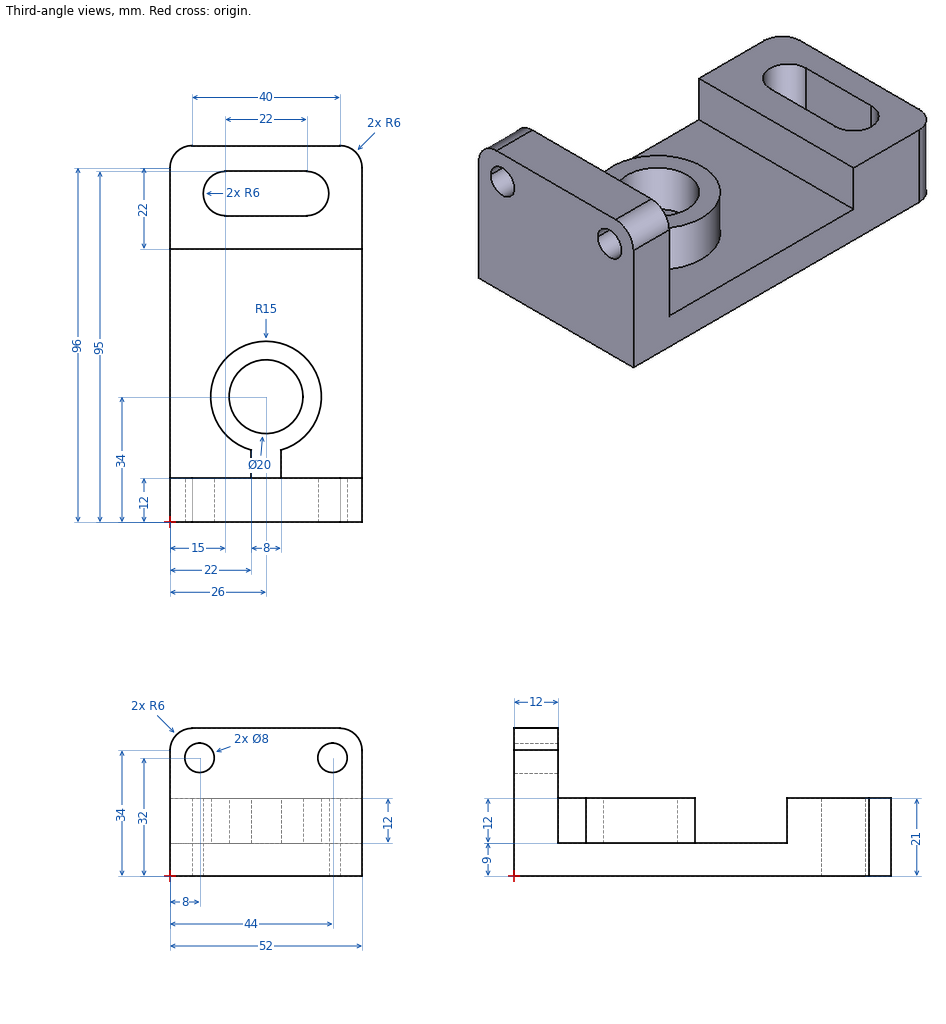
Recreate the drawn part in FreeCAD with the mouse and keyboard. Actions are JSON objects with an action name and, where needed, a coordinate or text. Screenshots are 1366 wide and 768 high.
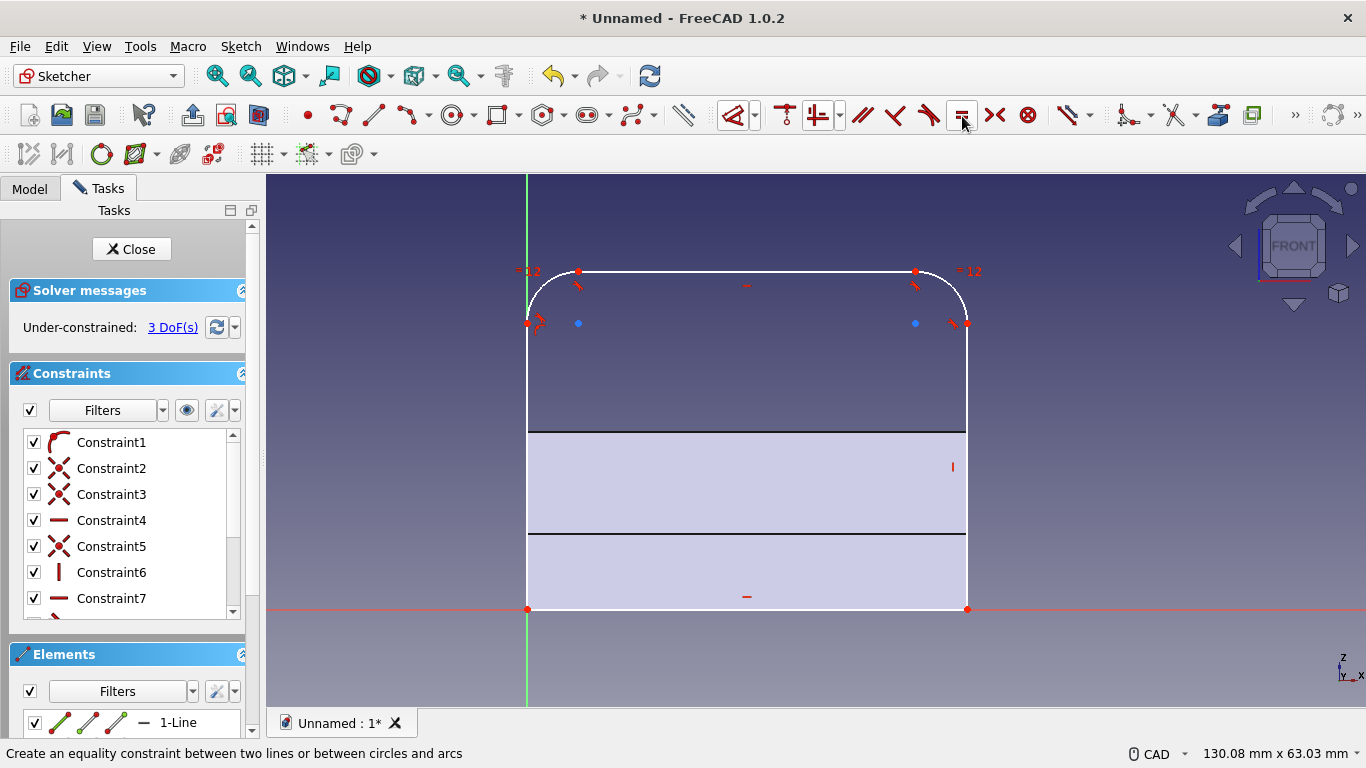
{"action": "left_click", "coordinate": [962, 300]}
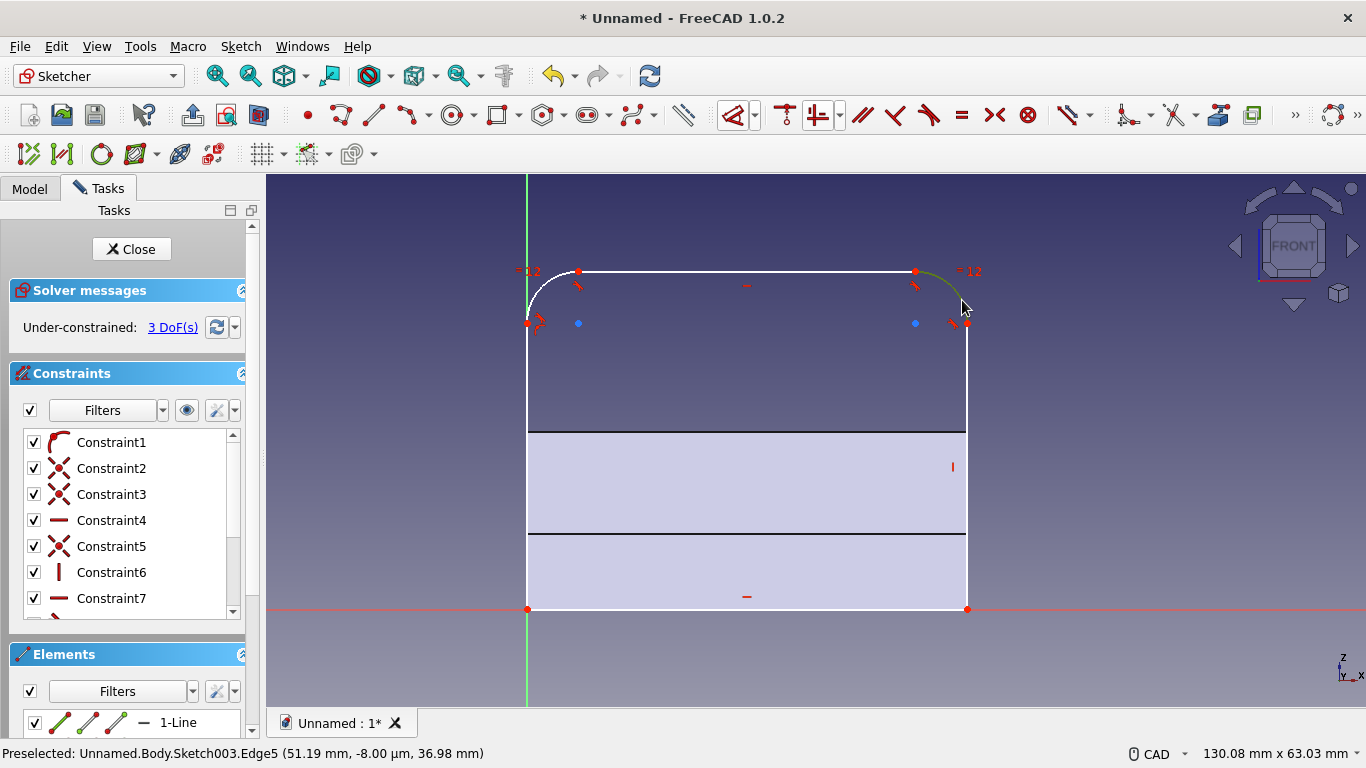
{"action": "left_click", "coordinate": [754, 116]}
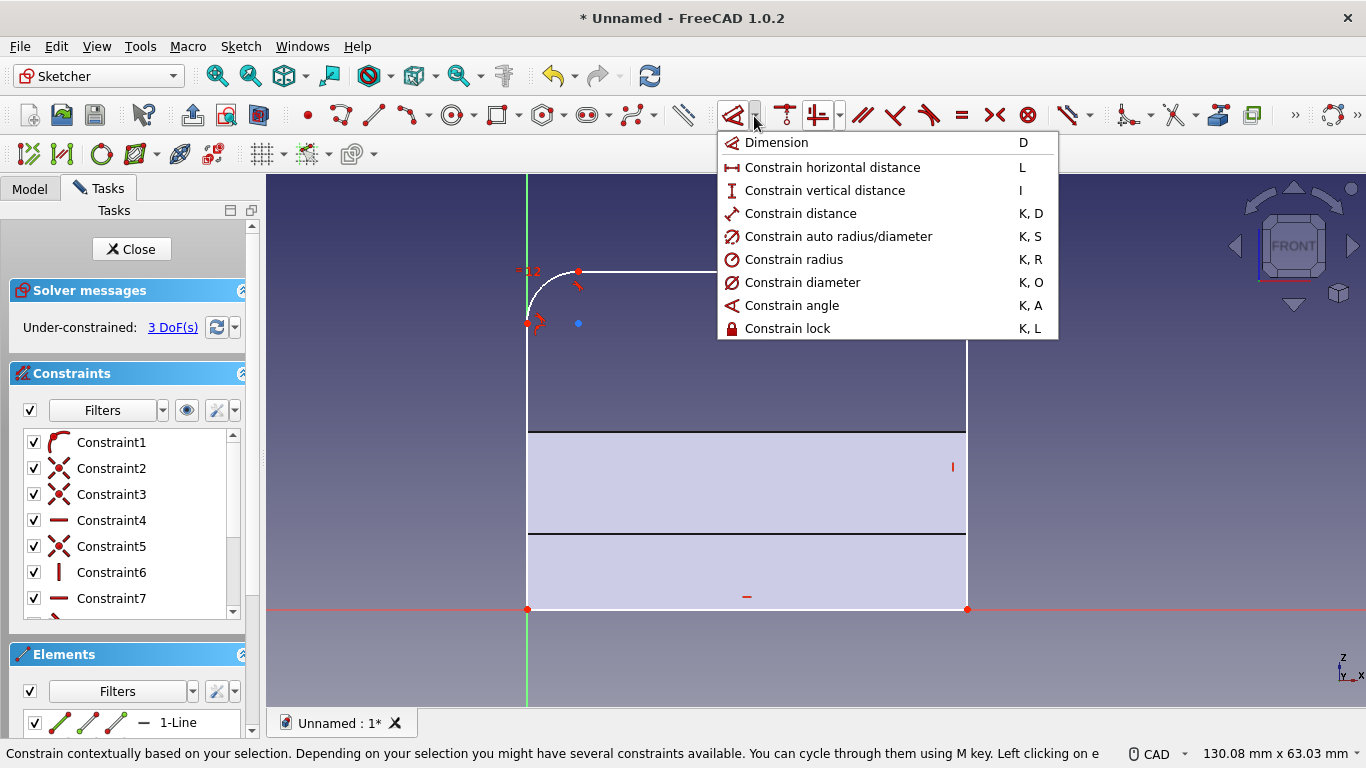
{"action": "left_click", "coordinate": [888, 260]}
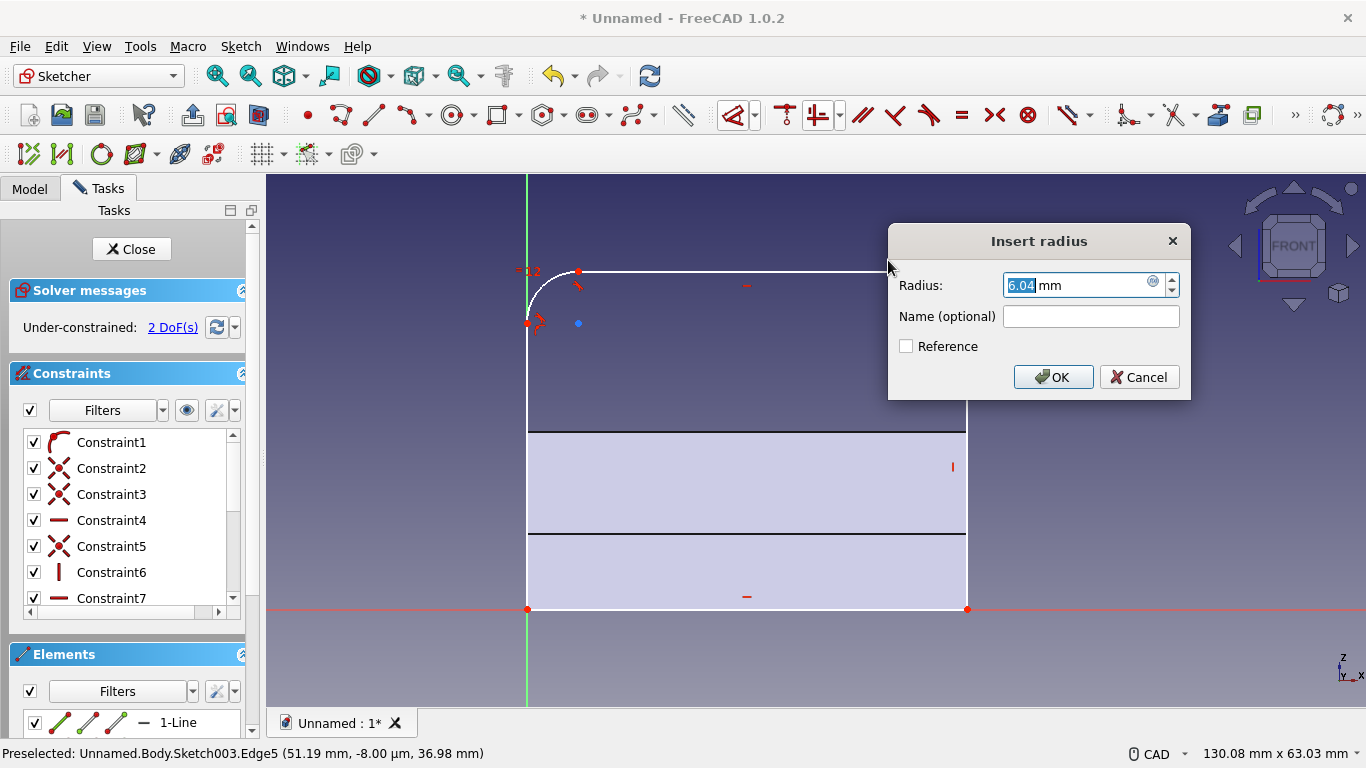
{"action": "type", "text": "6"}
{"action": "key", "text": "Return"}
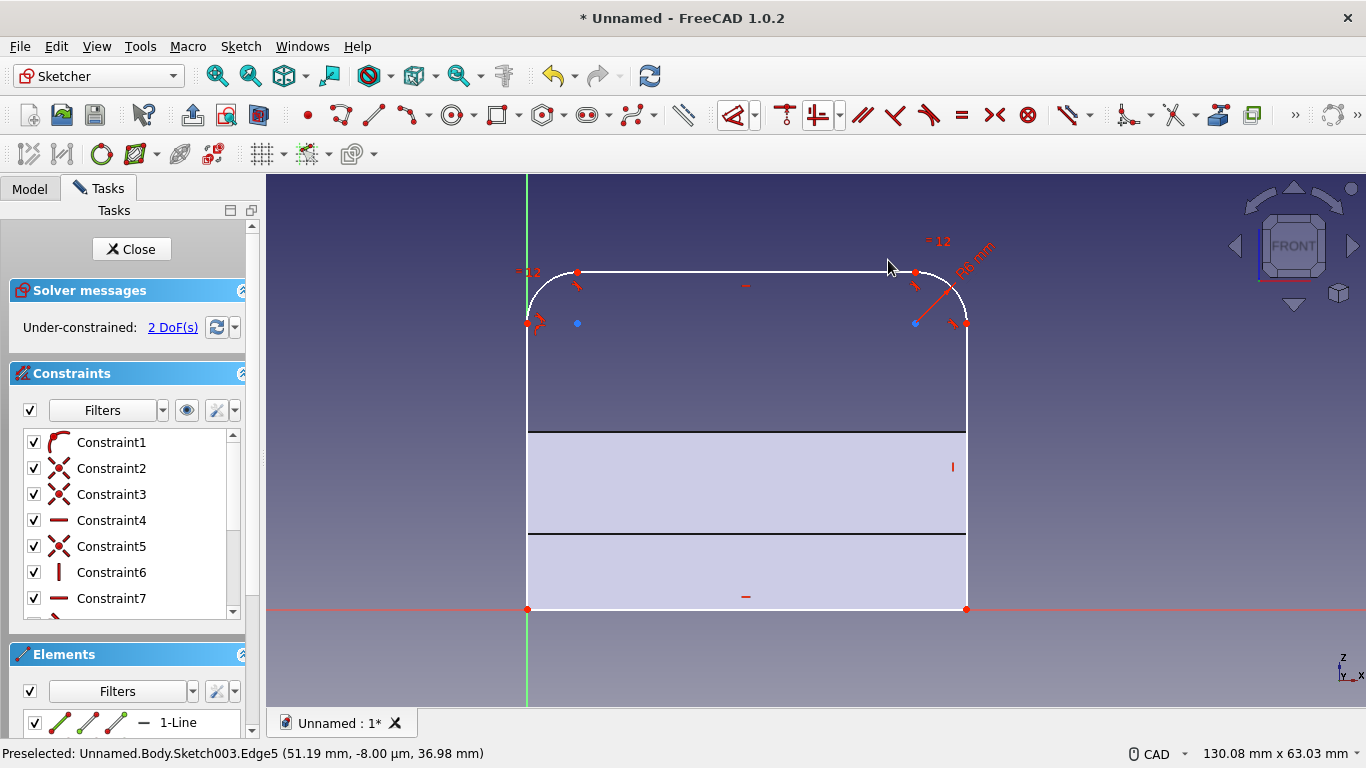
{"action": "left_click", "coordinate": [527, 409]}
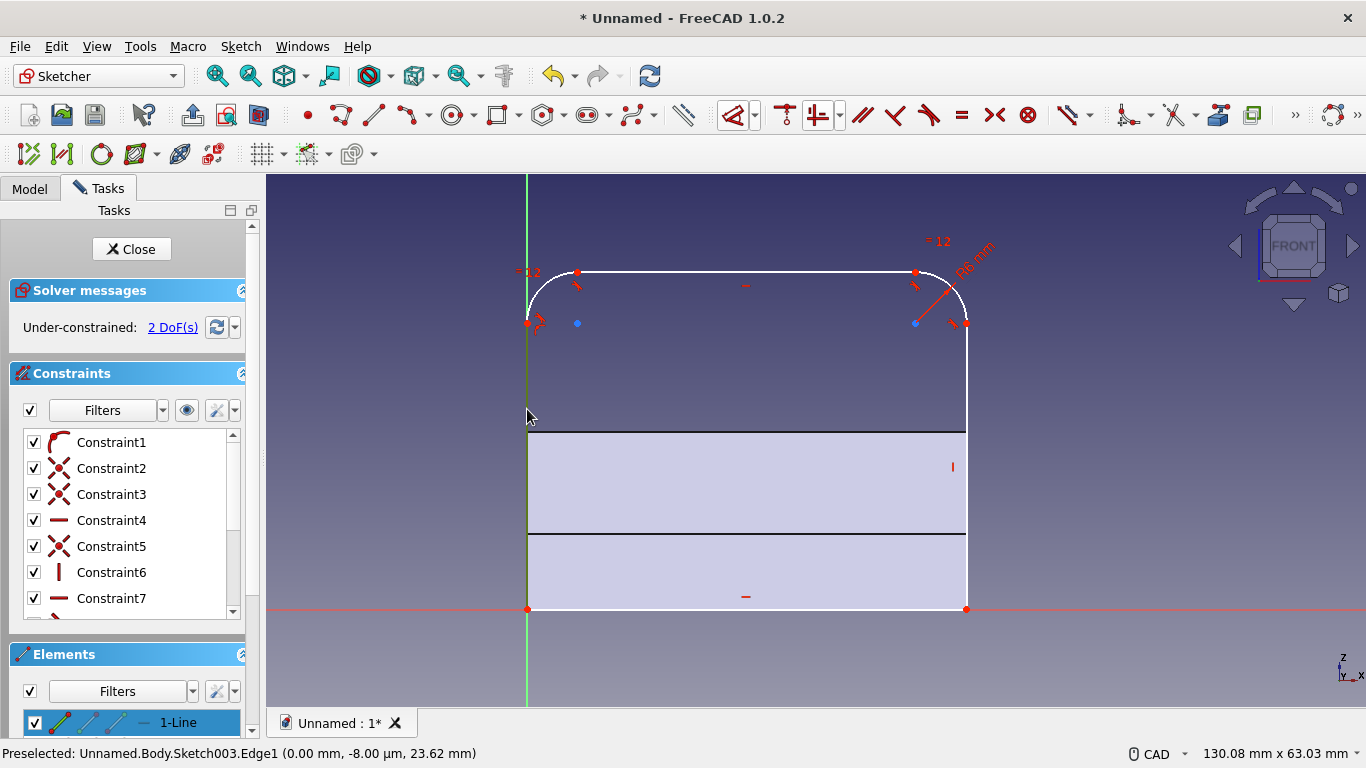
{"action": "key", "text": "i"}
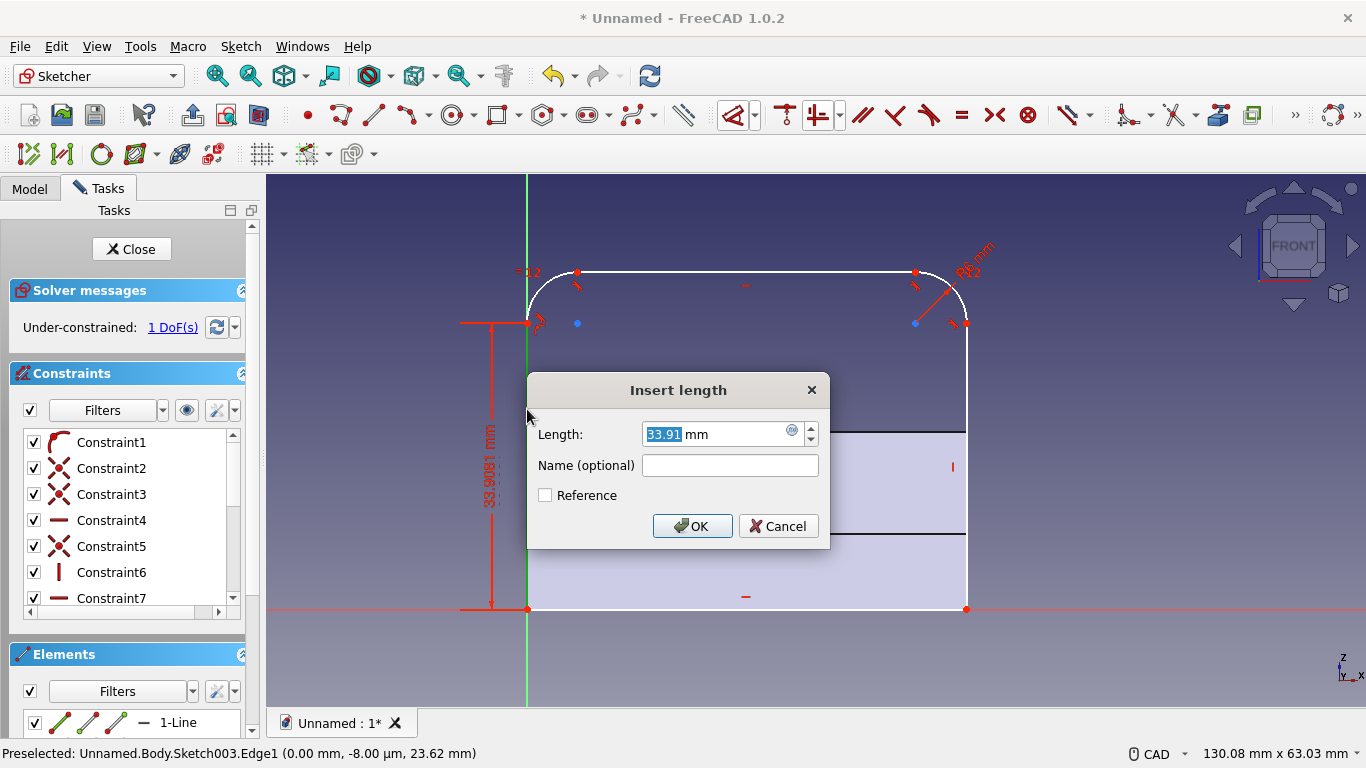
{"action": "type", "text": "34"}
{"action": "key", "text": "Return"}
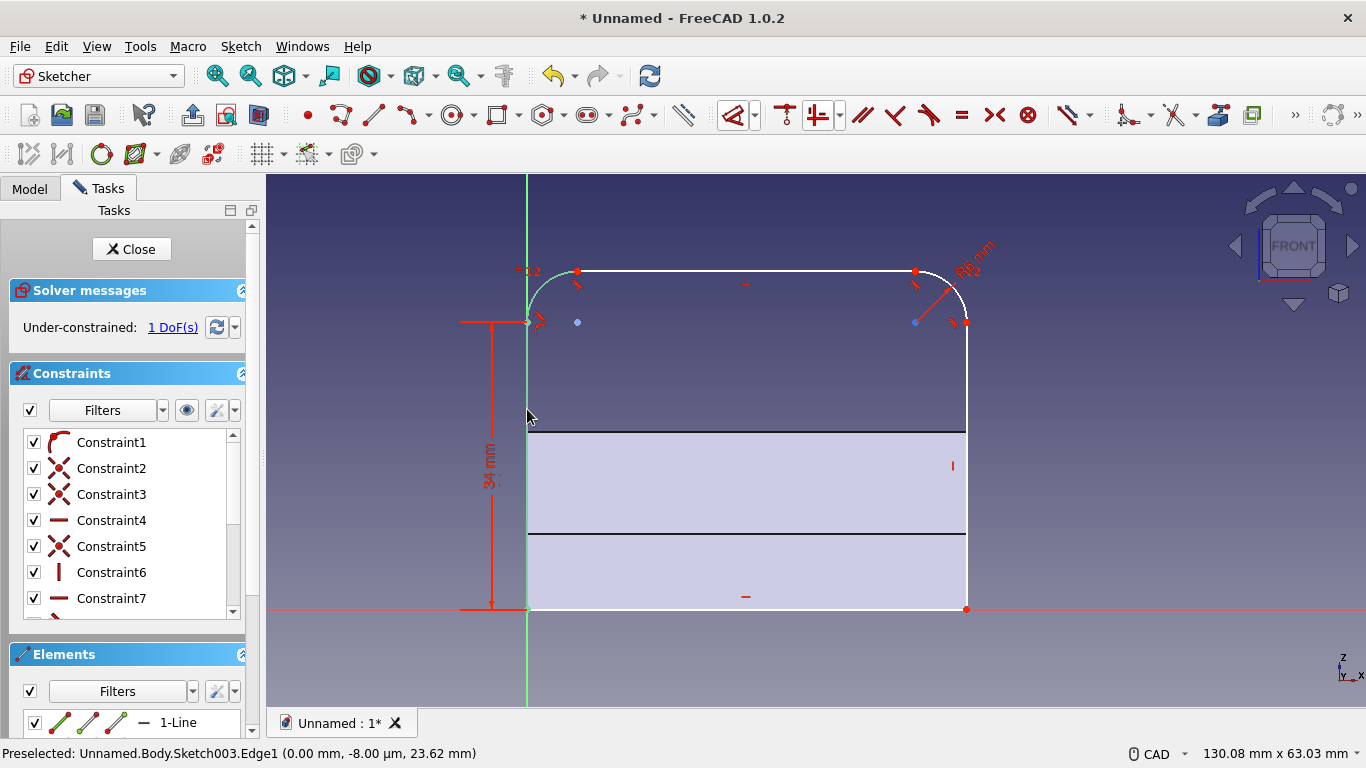
{"action": "left_click", "coordinate": [659, 610]}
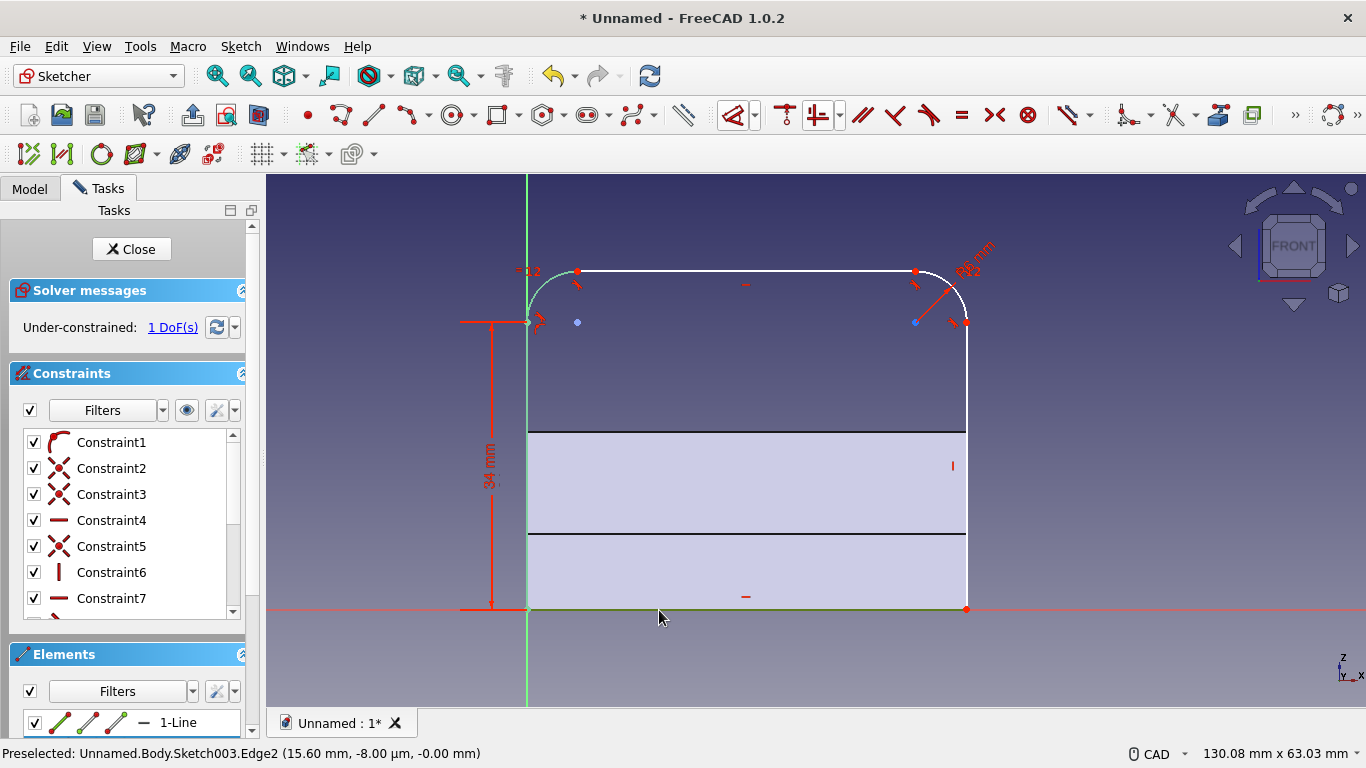
{"action": "left_click", "coordinate": [754, 116]}